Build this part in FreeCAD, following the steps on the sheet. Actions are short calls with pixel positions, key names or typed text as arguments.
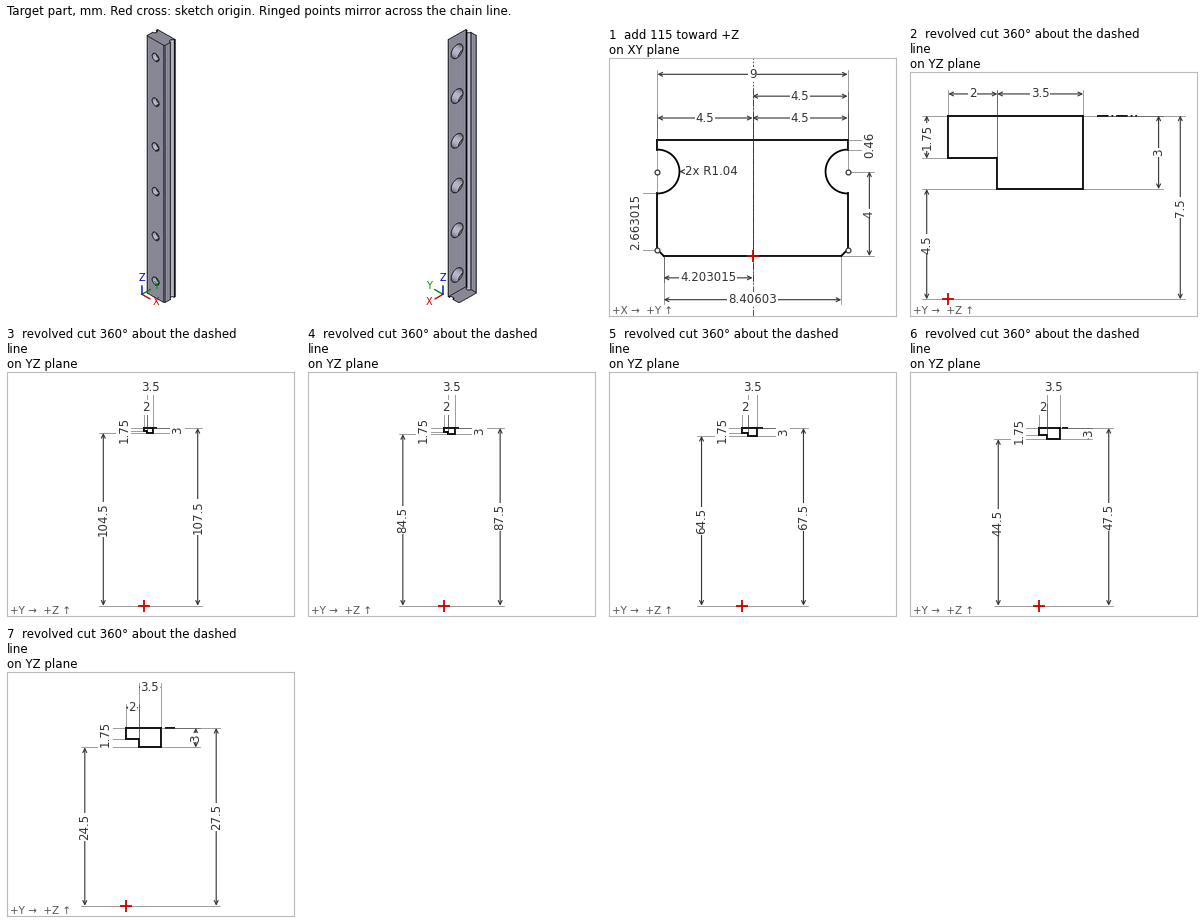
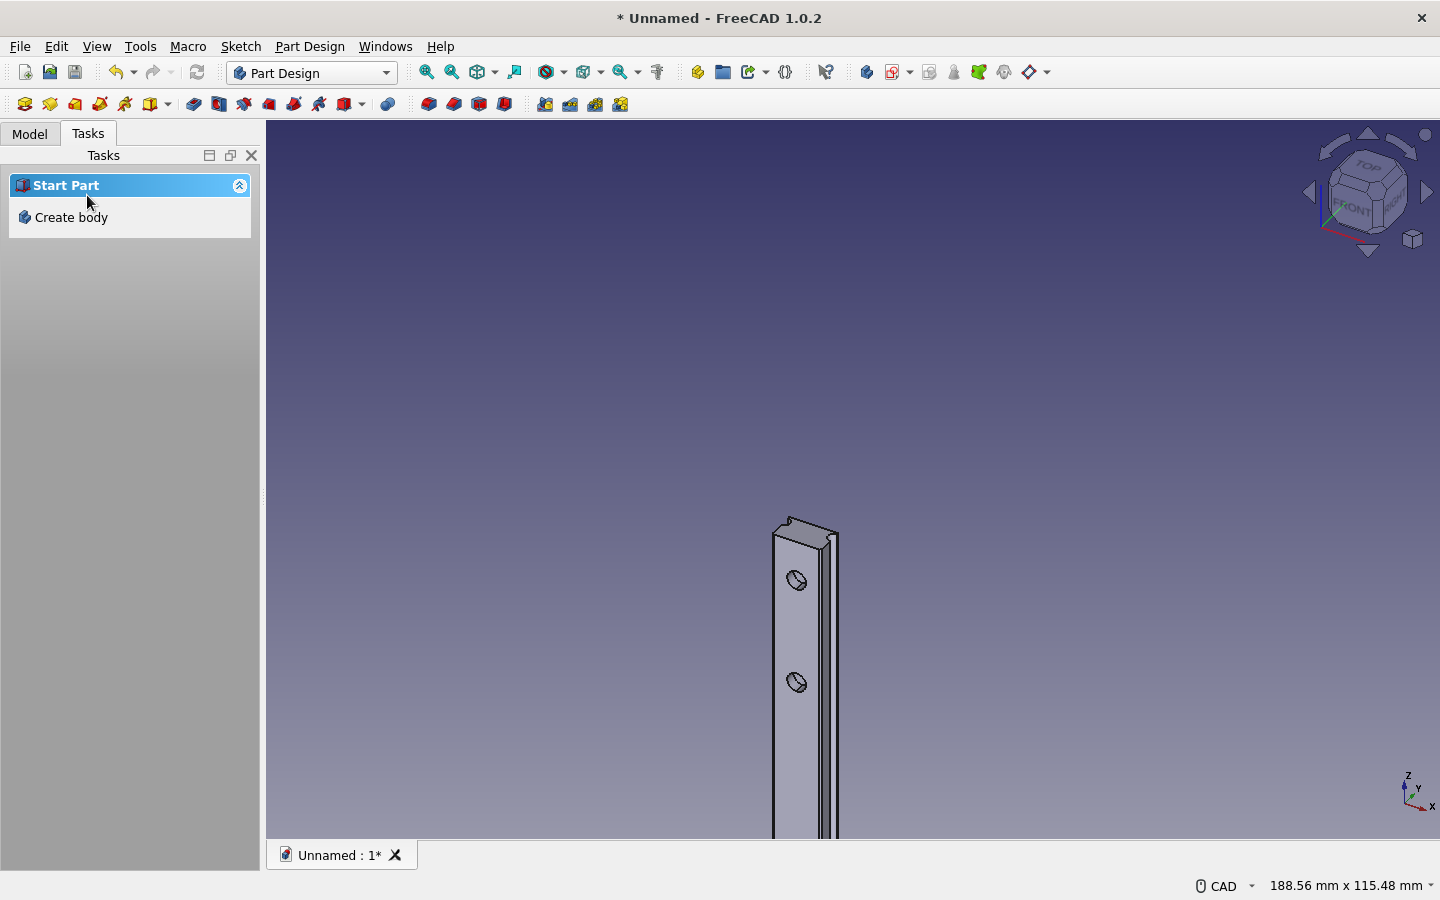
key(v)
key(f)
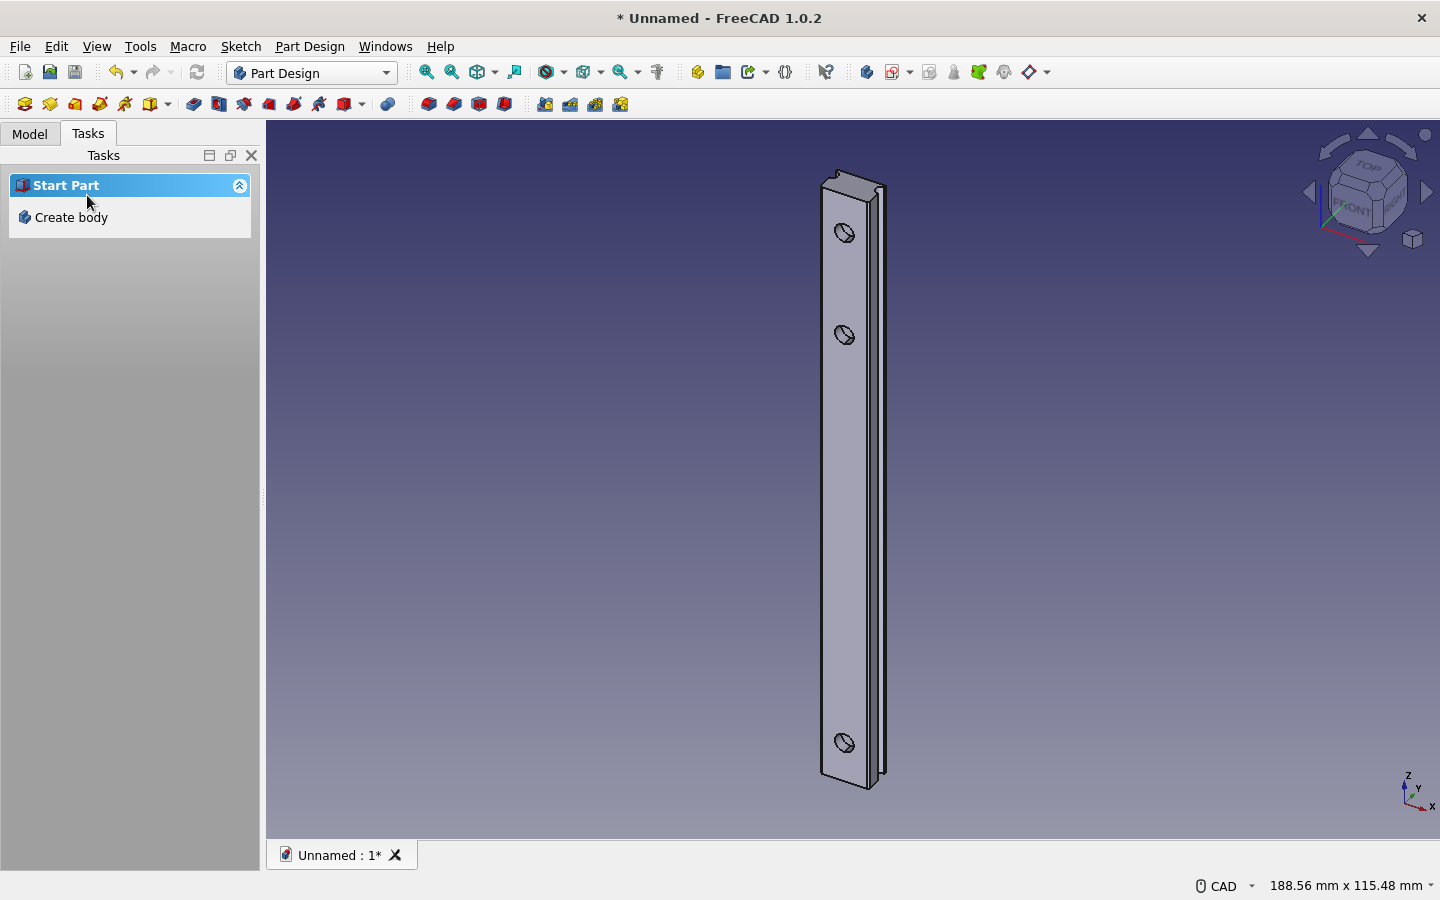
click(892, 72)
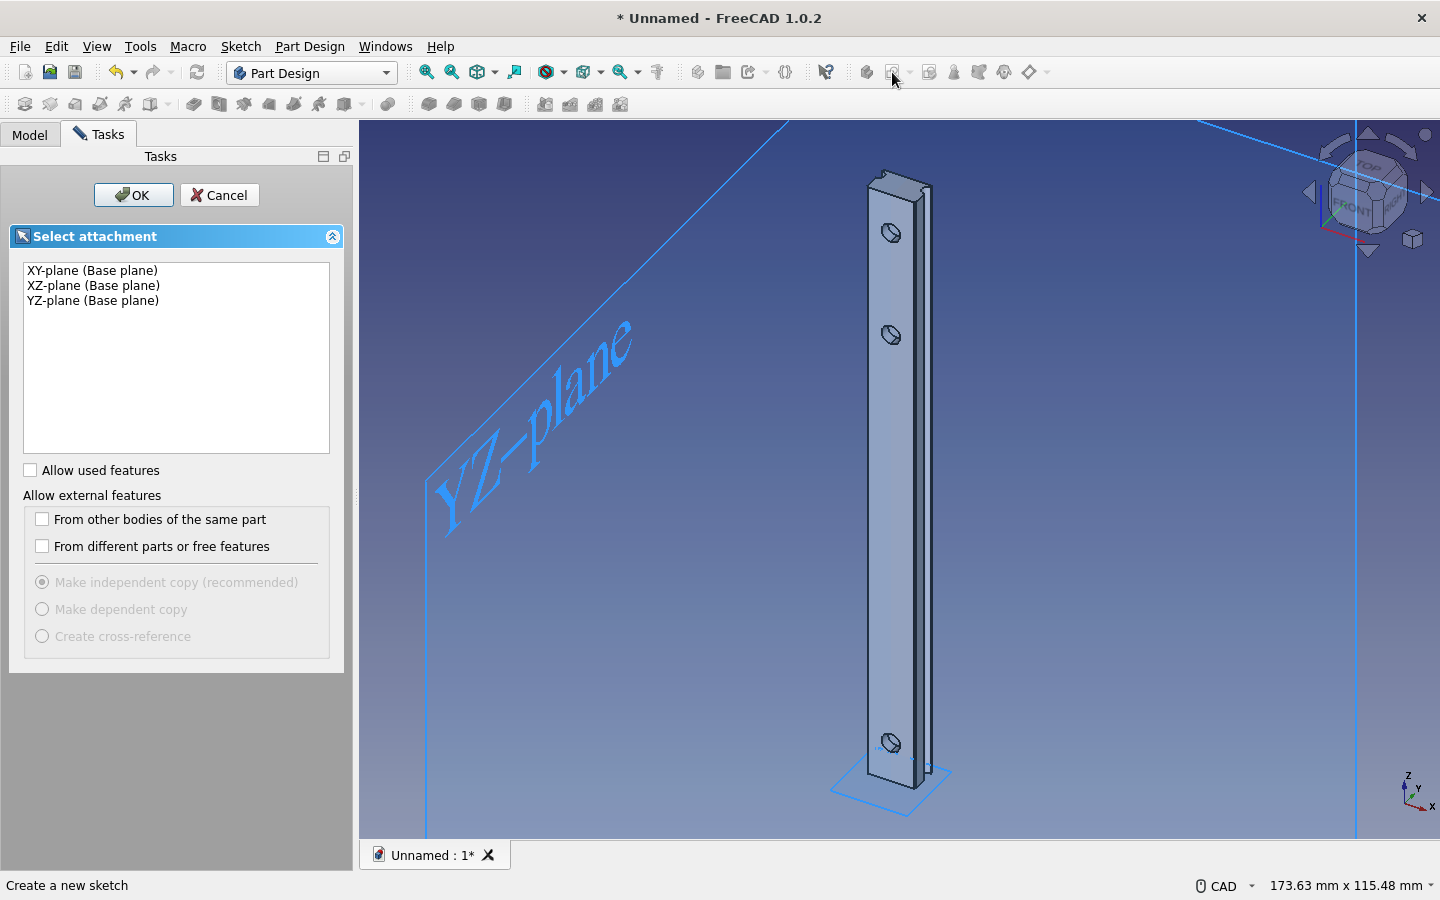
click(84, 300)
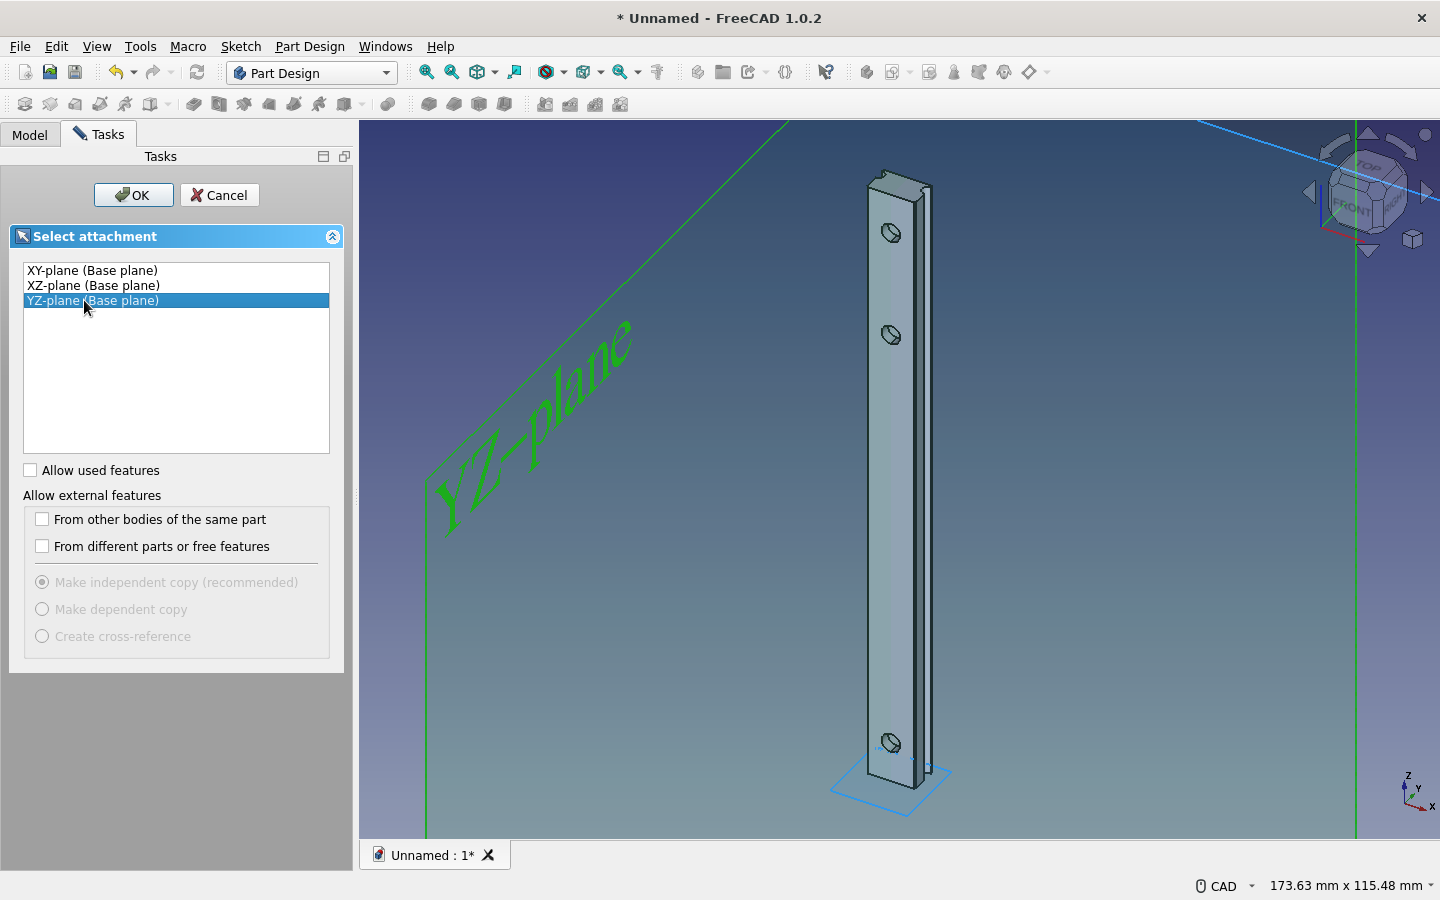
click(134, 195)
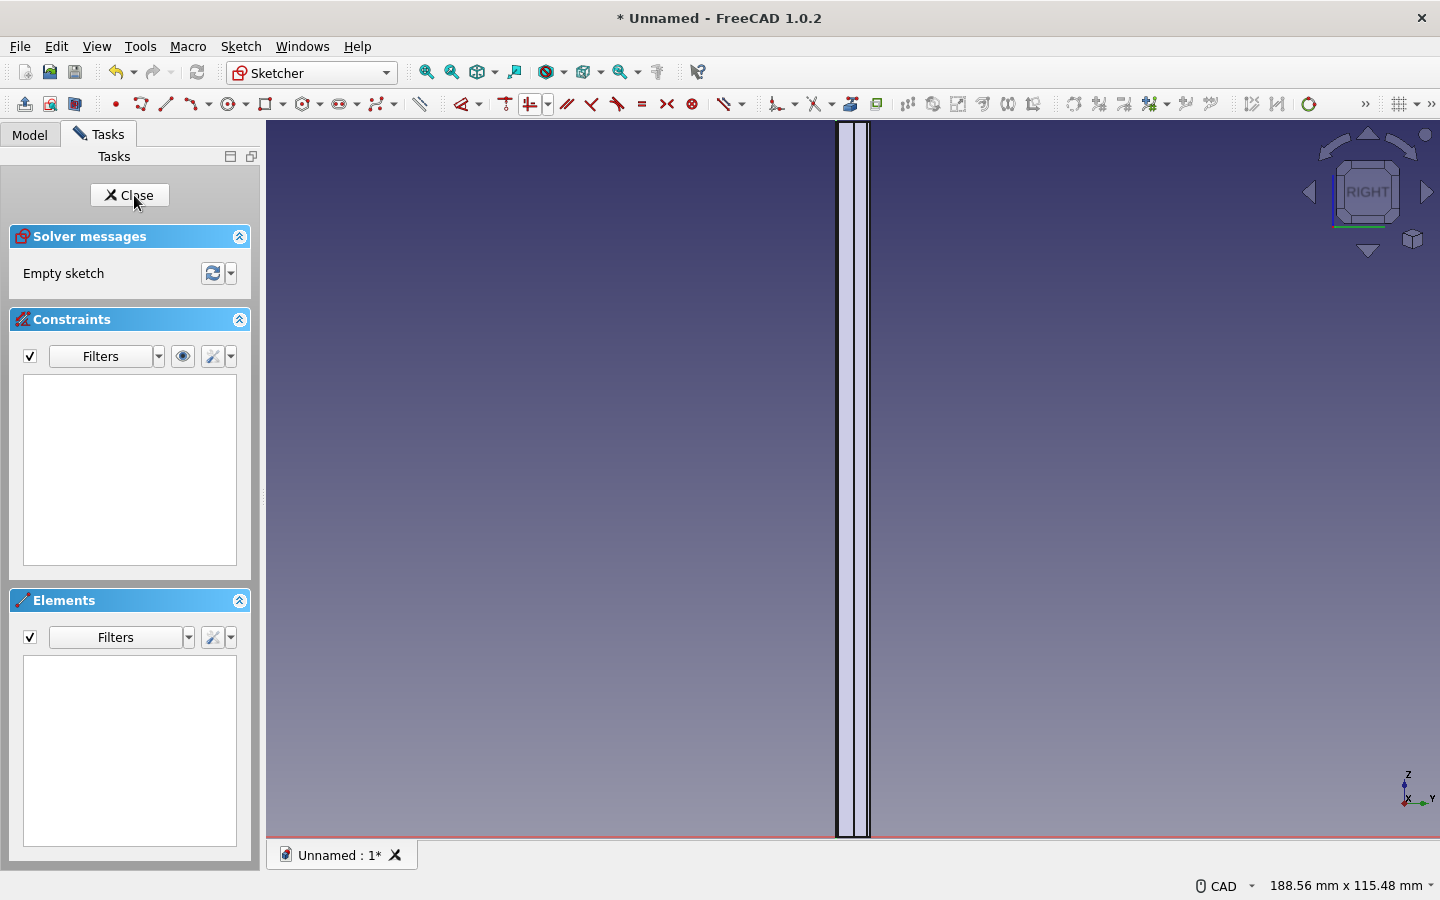
click(75, 104)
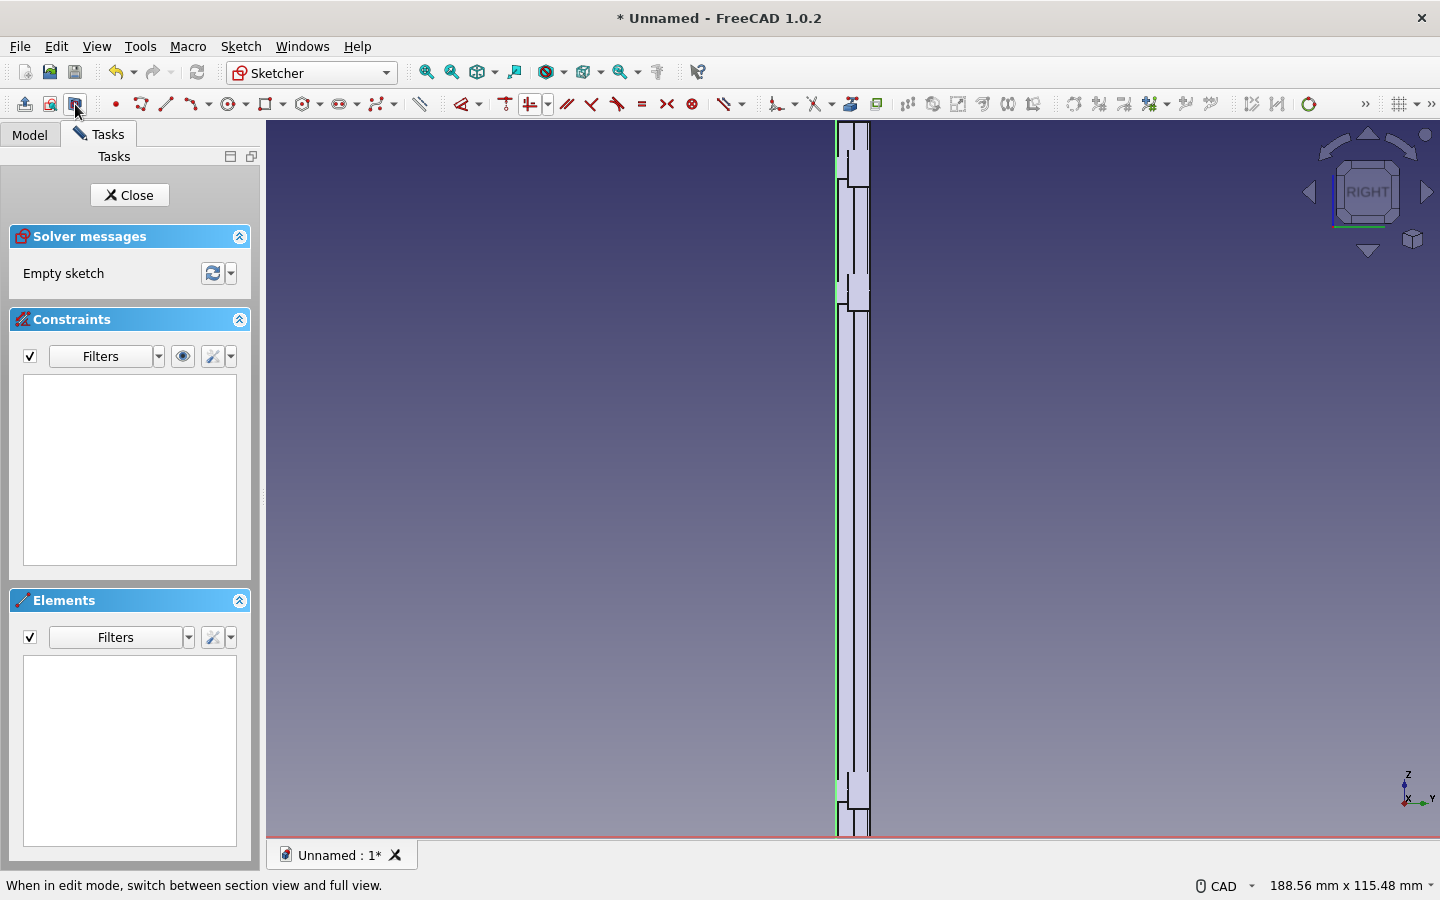
scroll(866, 422, up, 13)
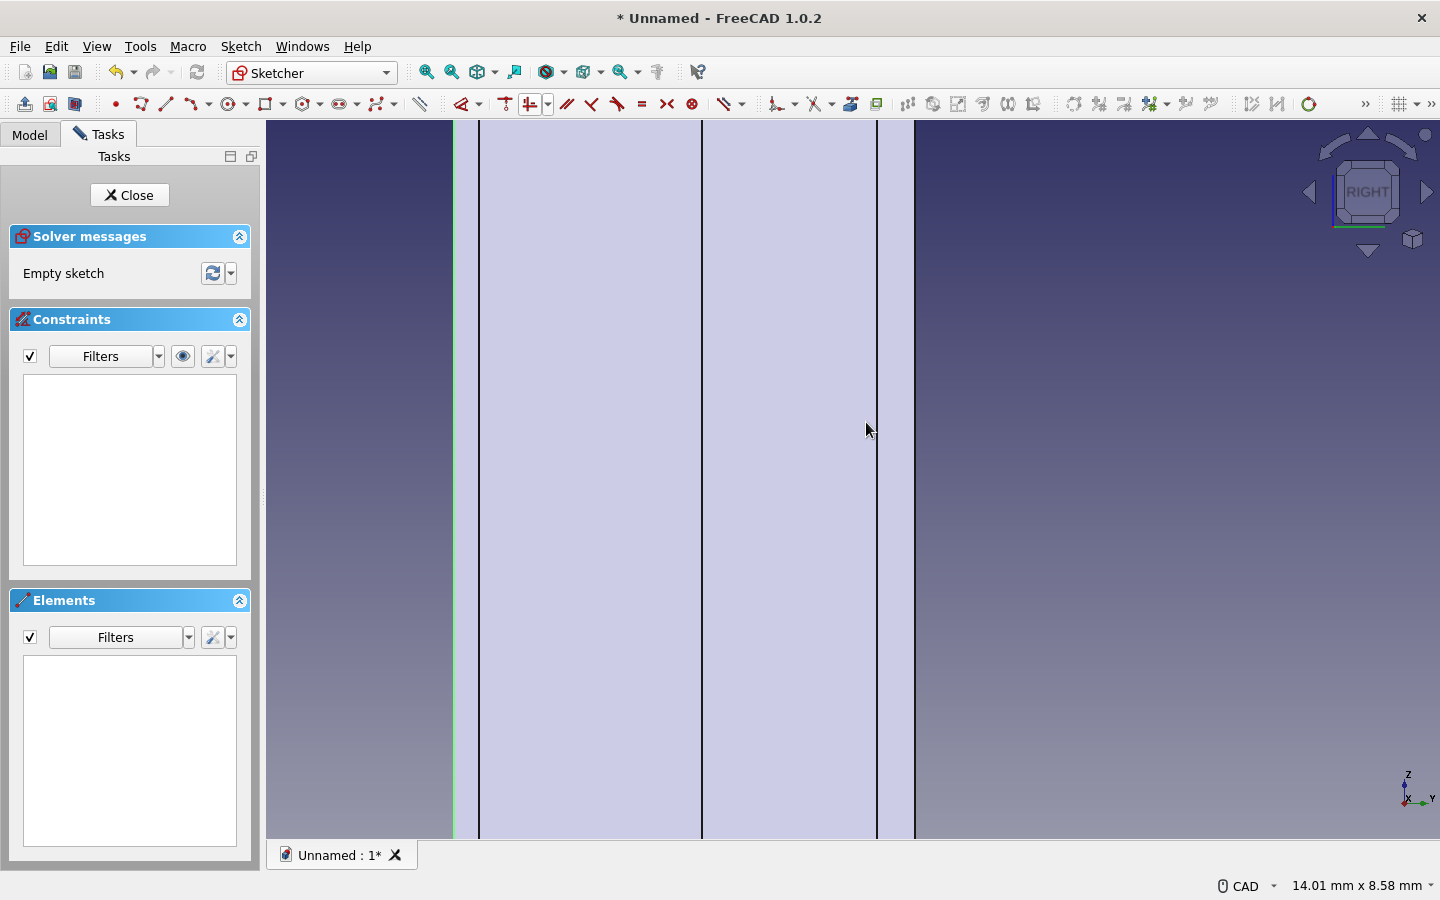
key(g)
key(m)